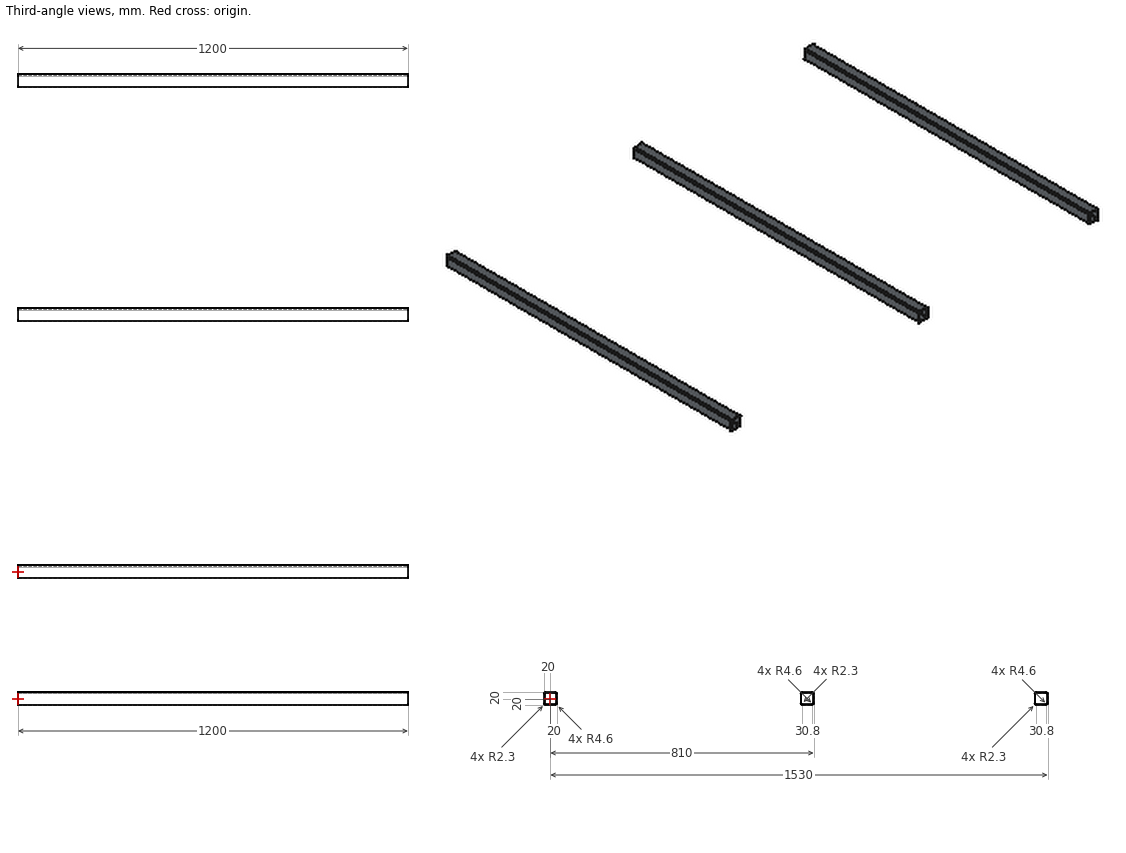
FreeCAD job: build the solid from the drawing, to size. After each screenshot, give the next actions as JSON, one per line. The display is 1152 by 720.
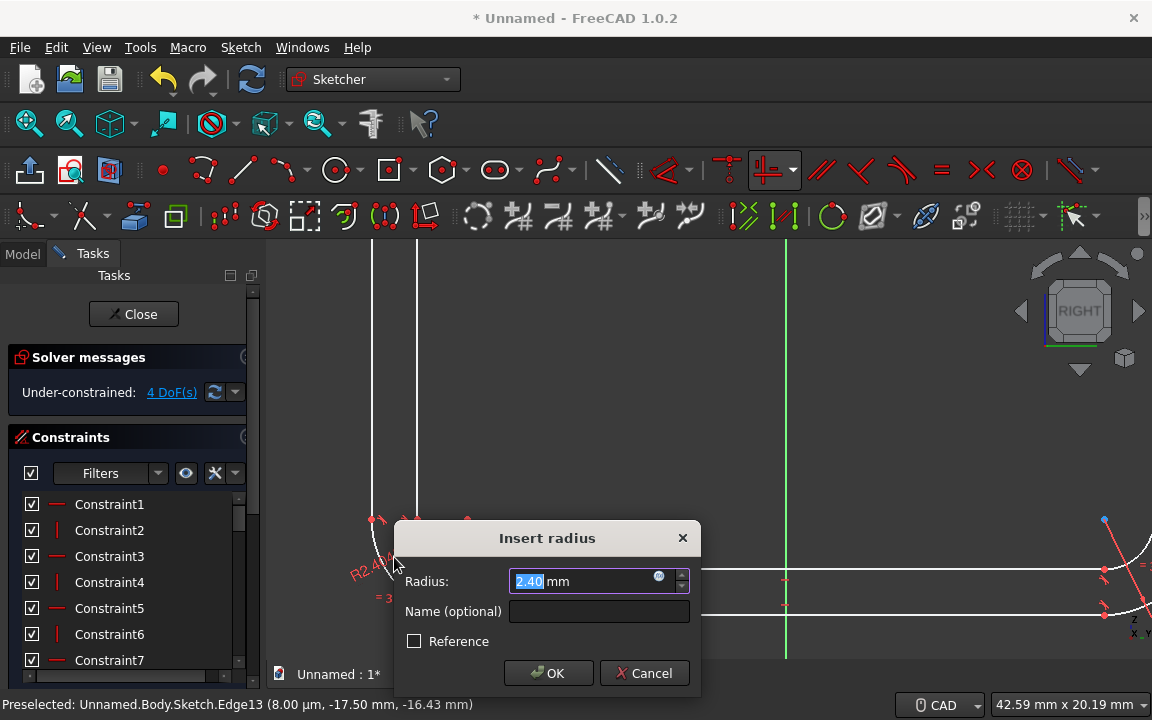
{"action": "type", "text": "2.3"}
{"action": "key", "text": "Return"}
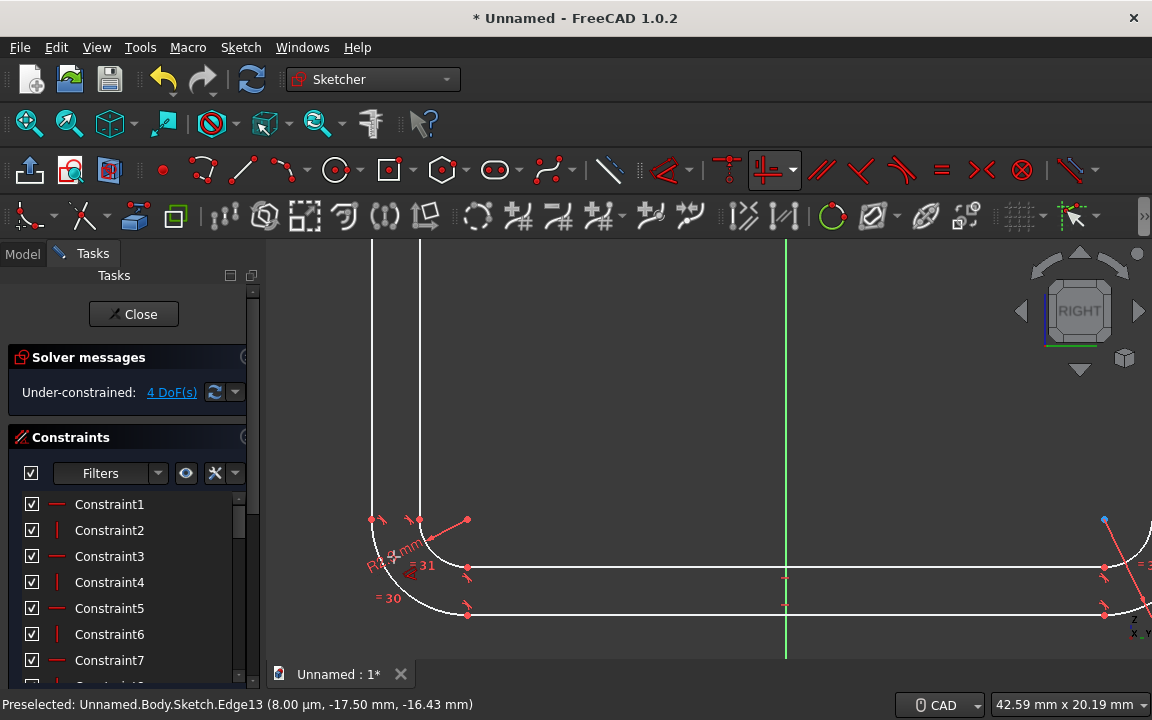
{"action": "left_click", "coordinate": [467, 615]}
{"action": "left_click", "coordinate": [433, 441]}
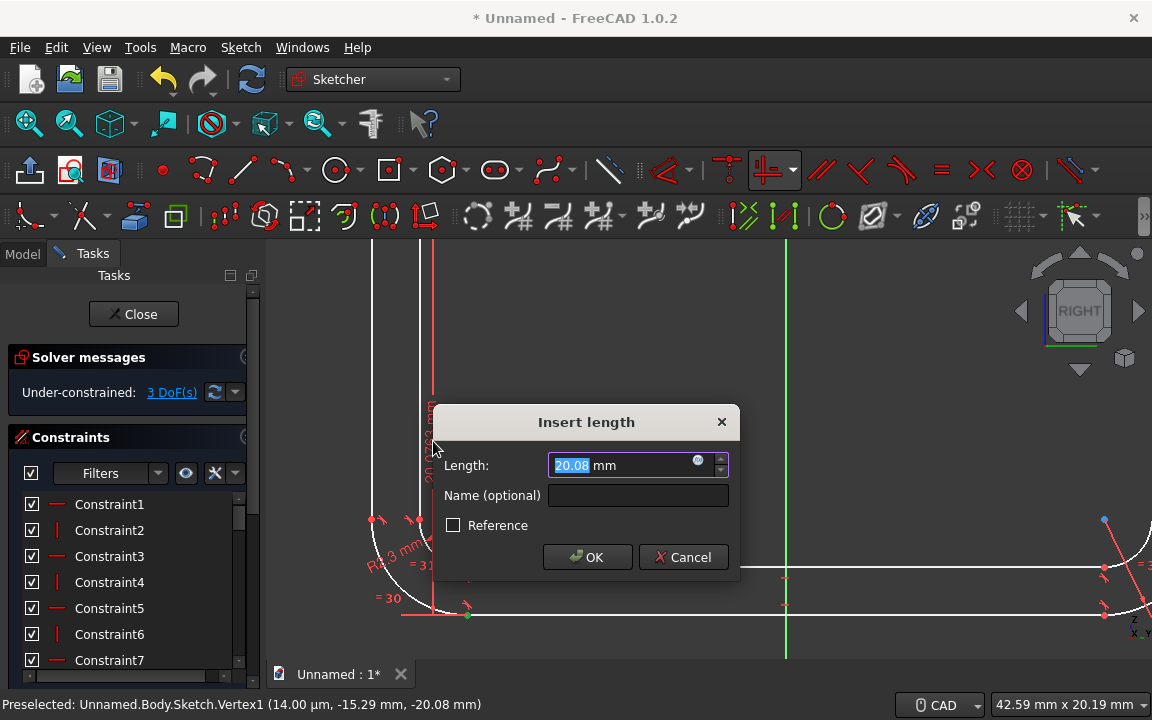
{"action": "type", "text": "20"}
{"action": "key", "text": "Return"}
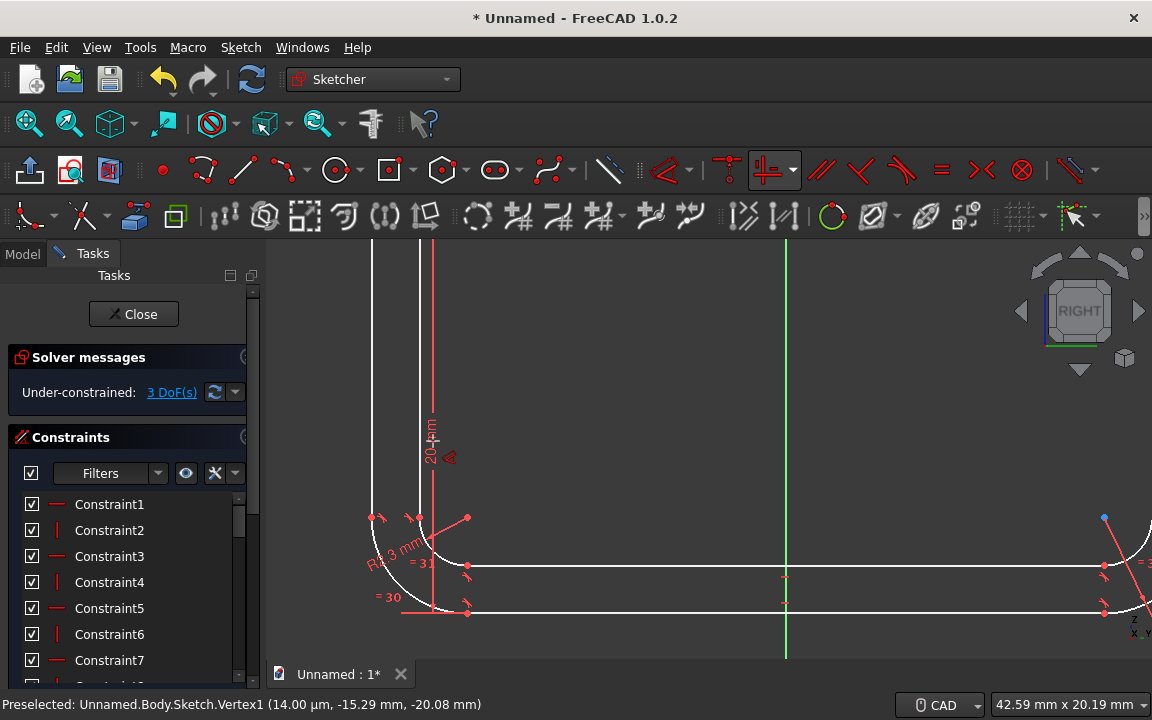
{"action": "scroll", "coordinate": [578, 557], "scroll_direction": "down", "scroll_amount": 6}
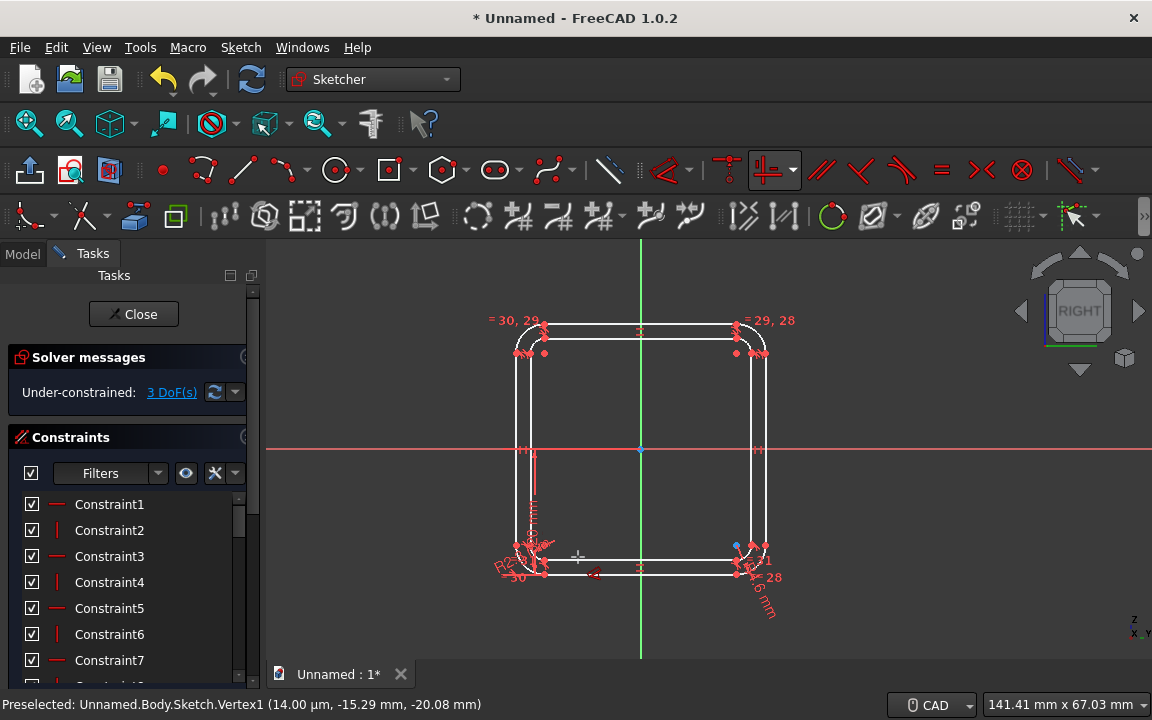
{"action": "left_click", "coordinate": [766, 546]}
{"action": "left_click", "coordinate": [703, 415]}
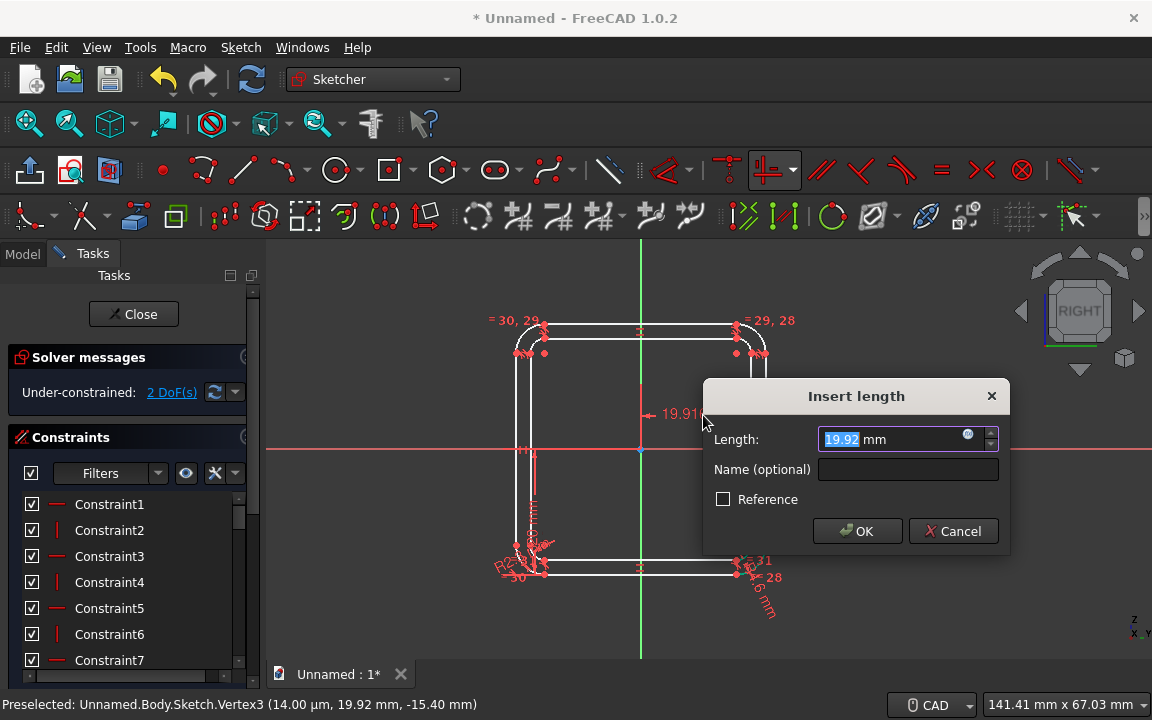
{"action": "type", "text": "20"}
{"action": "key", "text": "Return"}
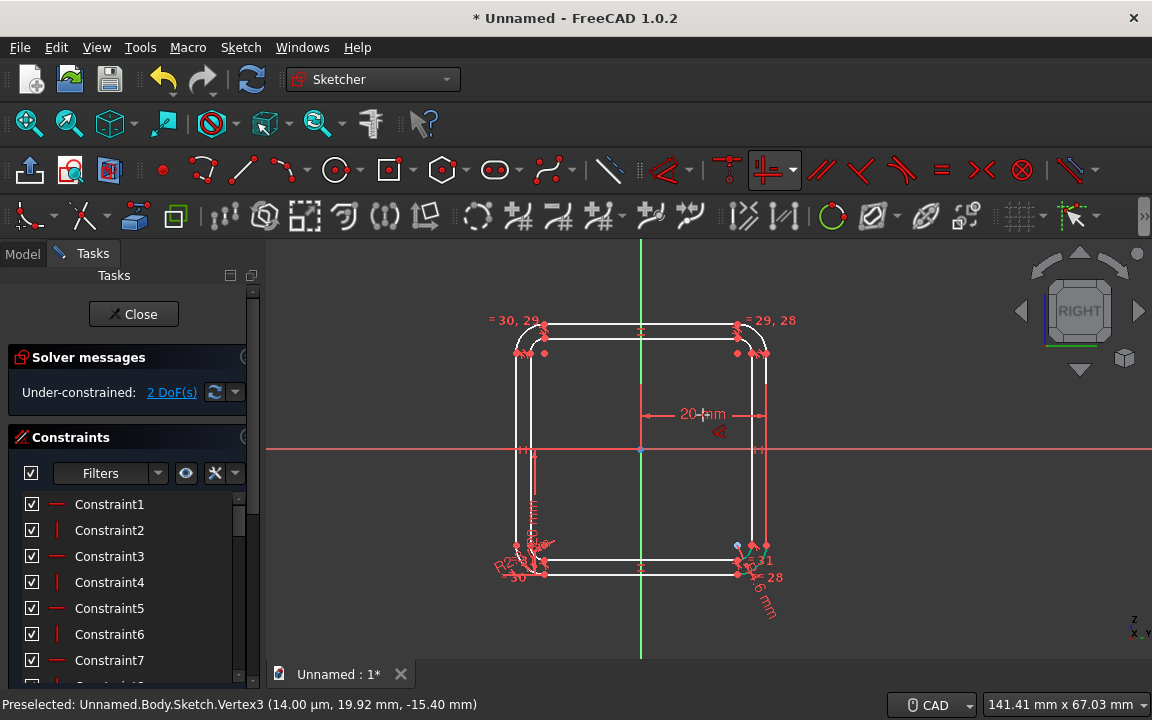
{"action": "left_click", "coordinate": [737, 324]}
{"action": "left_click", "coordinate": [607, 387]}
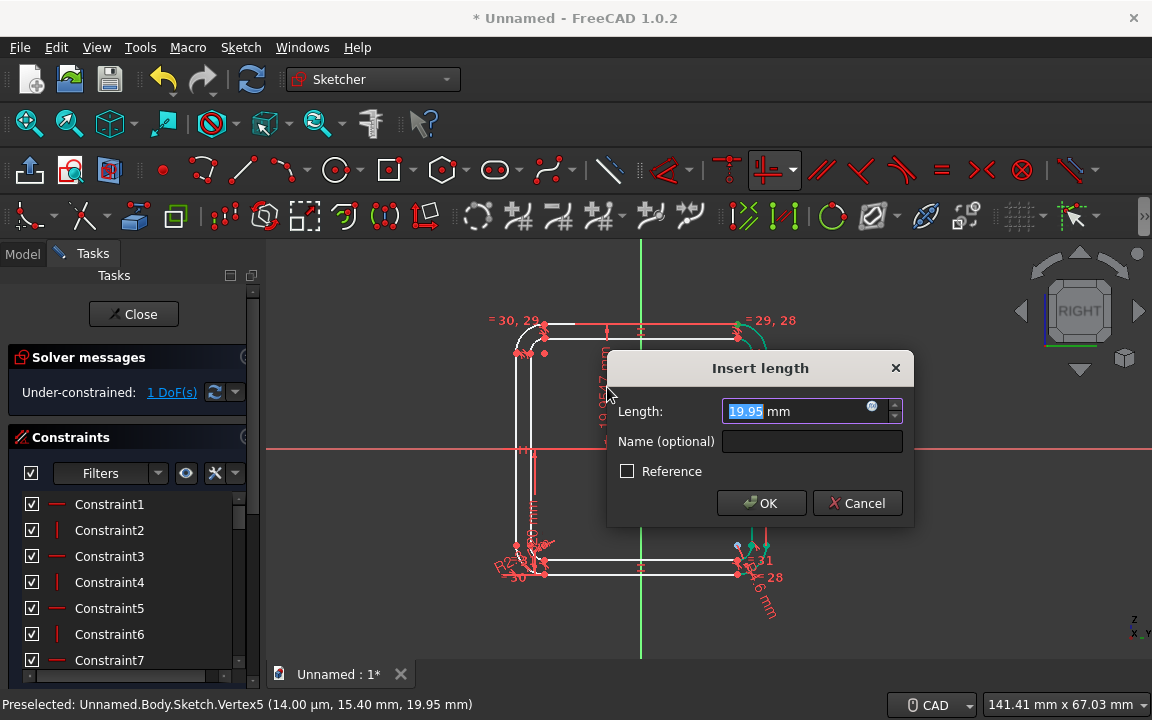
{"action": "type", "text": "20"}
{"action": "key", "text": "Return"}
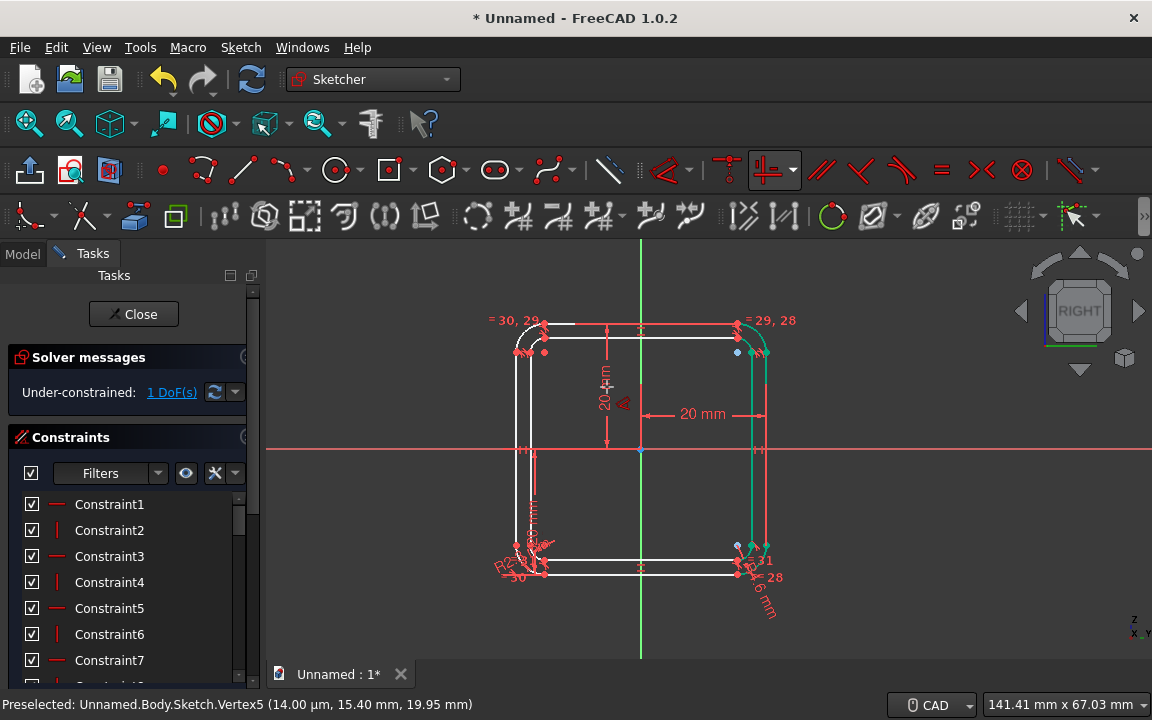
{"action": "left_click", "coordinate": [516, 353]}
{"action": "left_click", "coordinate": [578, 483]}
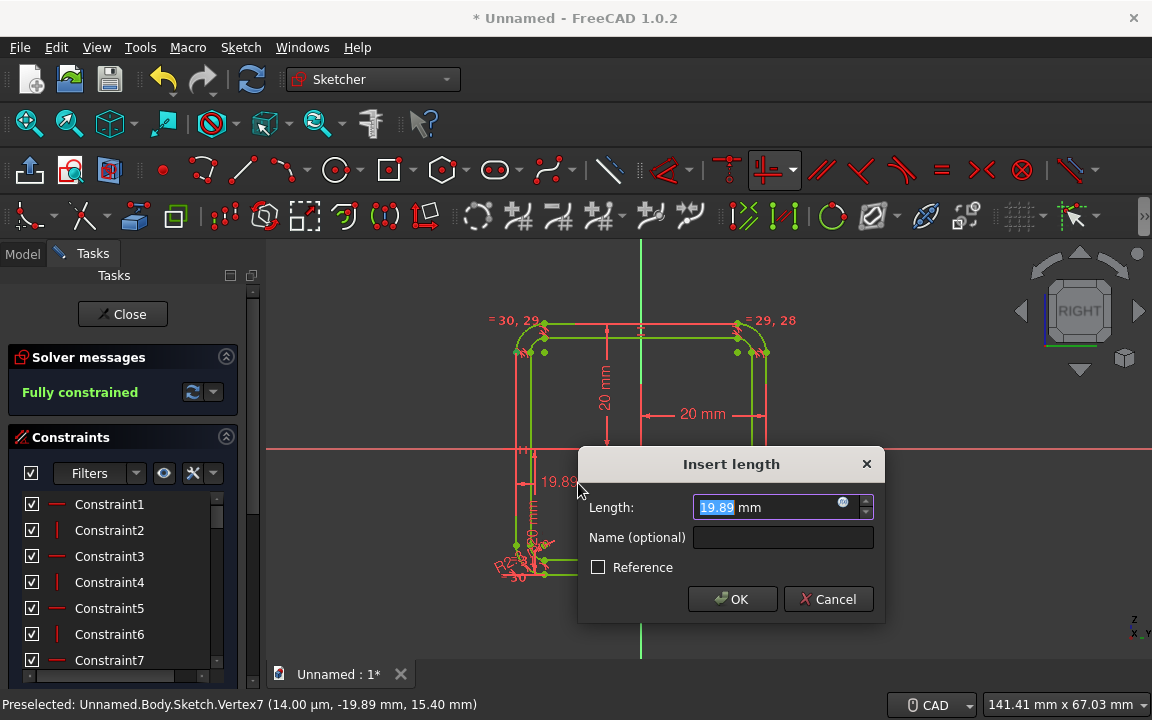
{"action": "type", "text": "20"}
{"action": "key", "text": "Return"}
{"action": "key", "text": "Escape"}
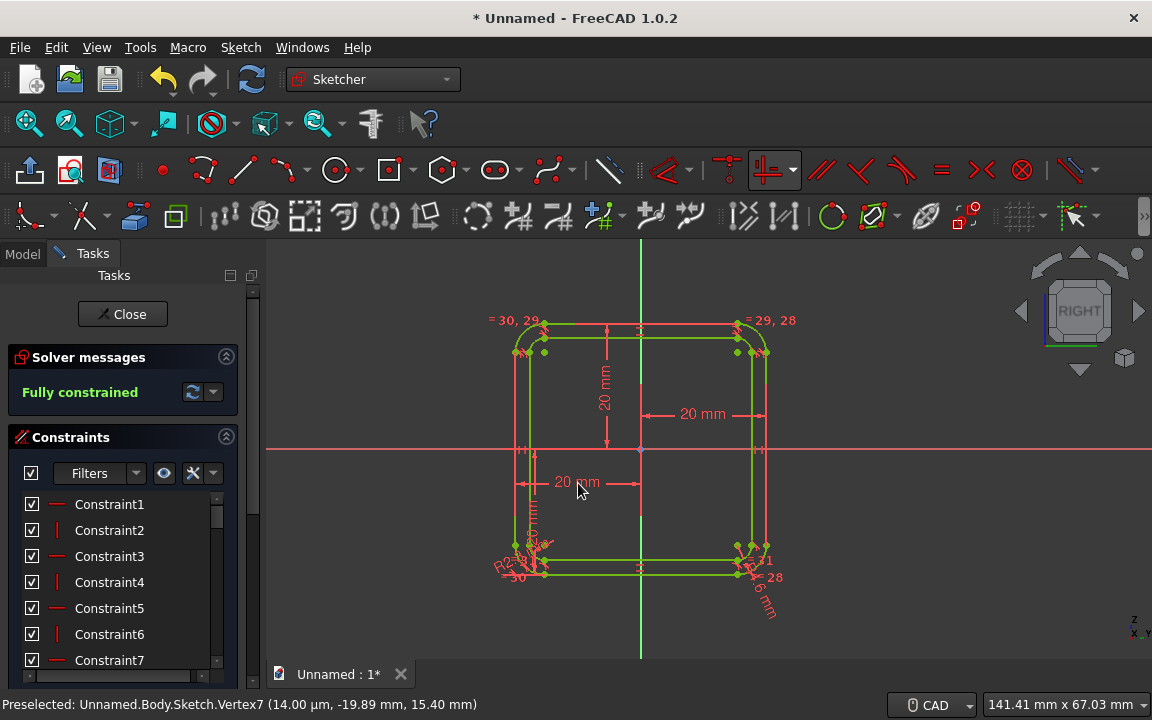
{"action": "left_click", "coordinate": [123, 314]}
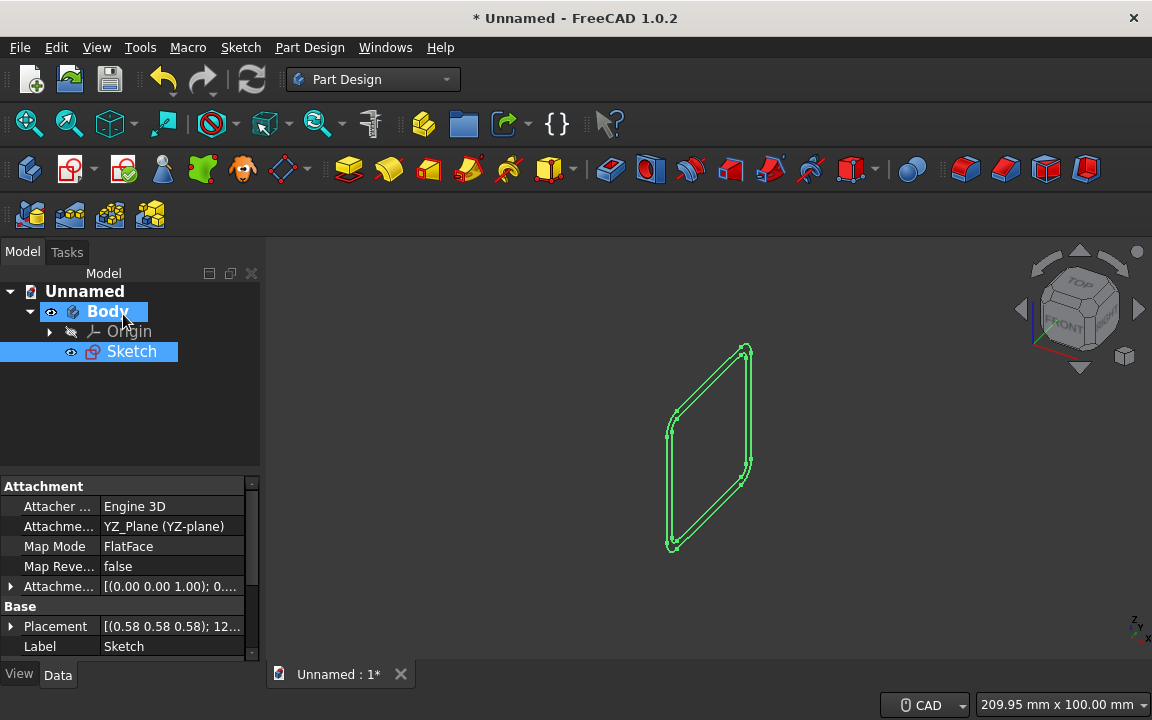
{"action": "left_click", "coordinate": [350, 170]}